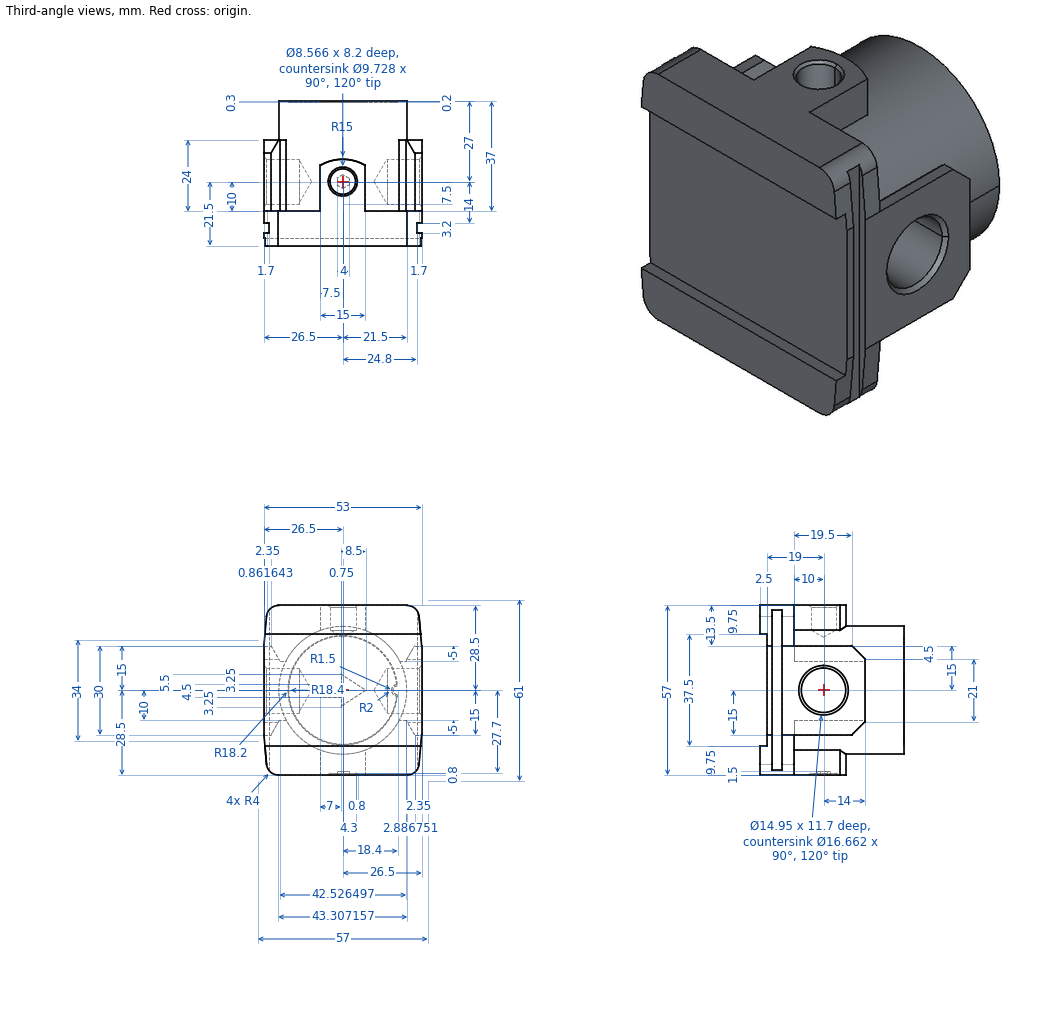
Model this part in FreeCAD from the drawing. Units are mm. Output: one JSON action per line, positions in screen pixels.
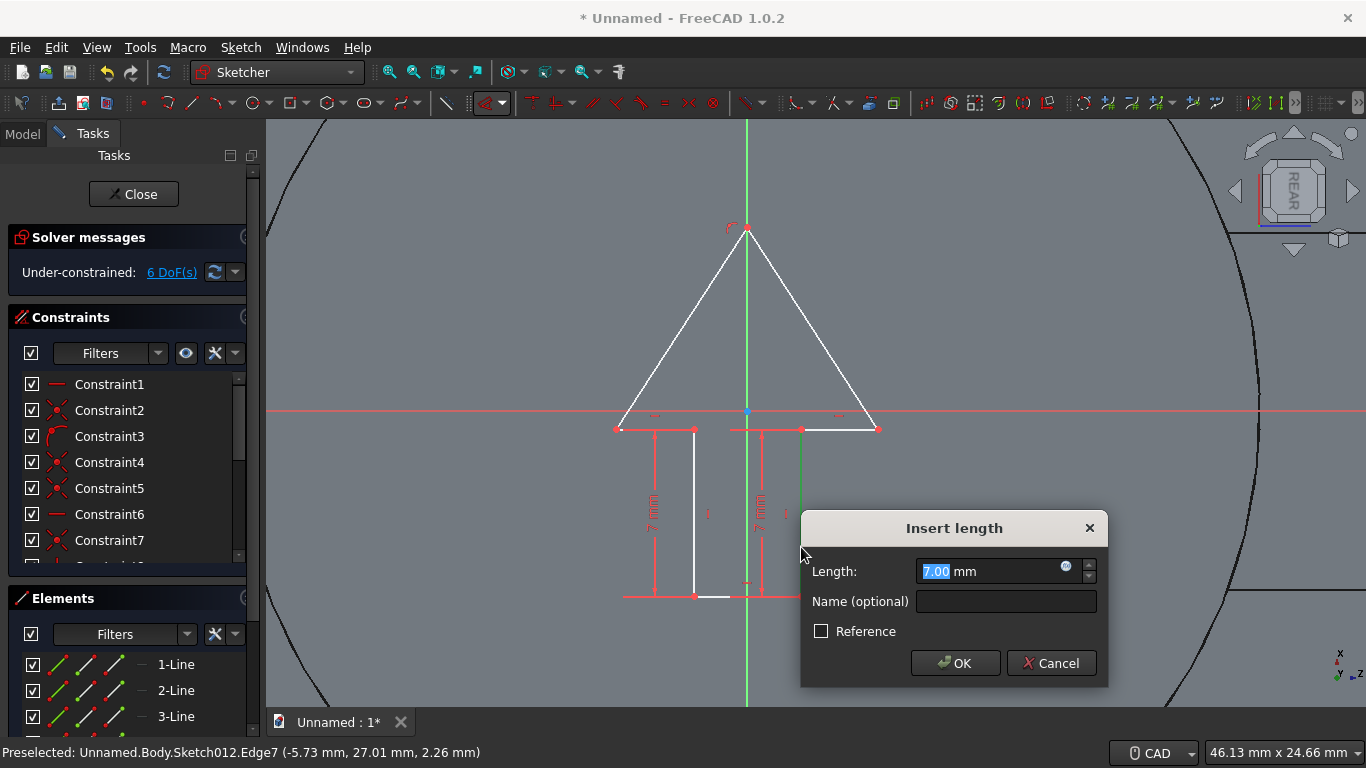
{"action": "type", "text": "7"}
{"action": "key", "text": "Return"}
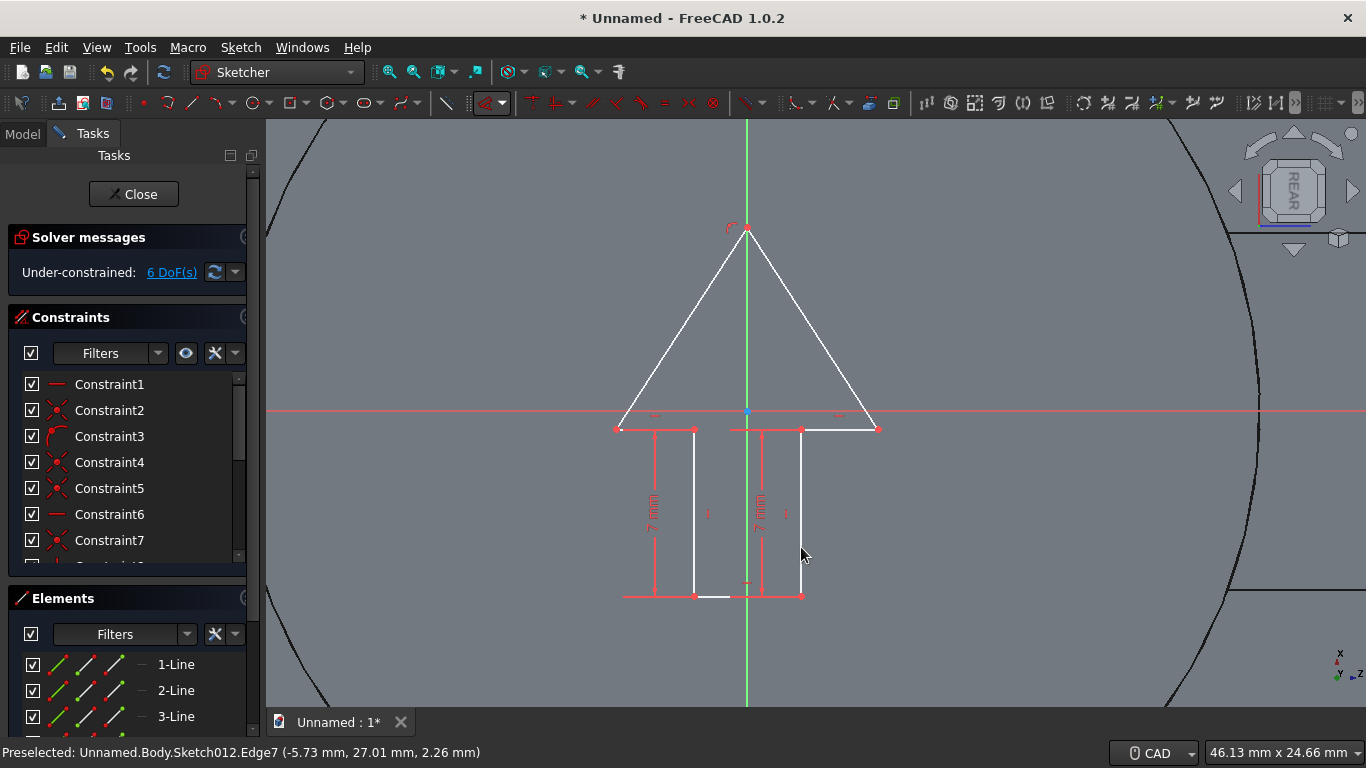
{"action": "left_click", "coordinate": [726, 597]}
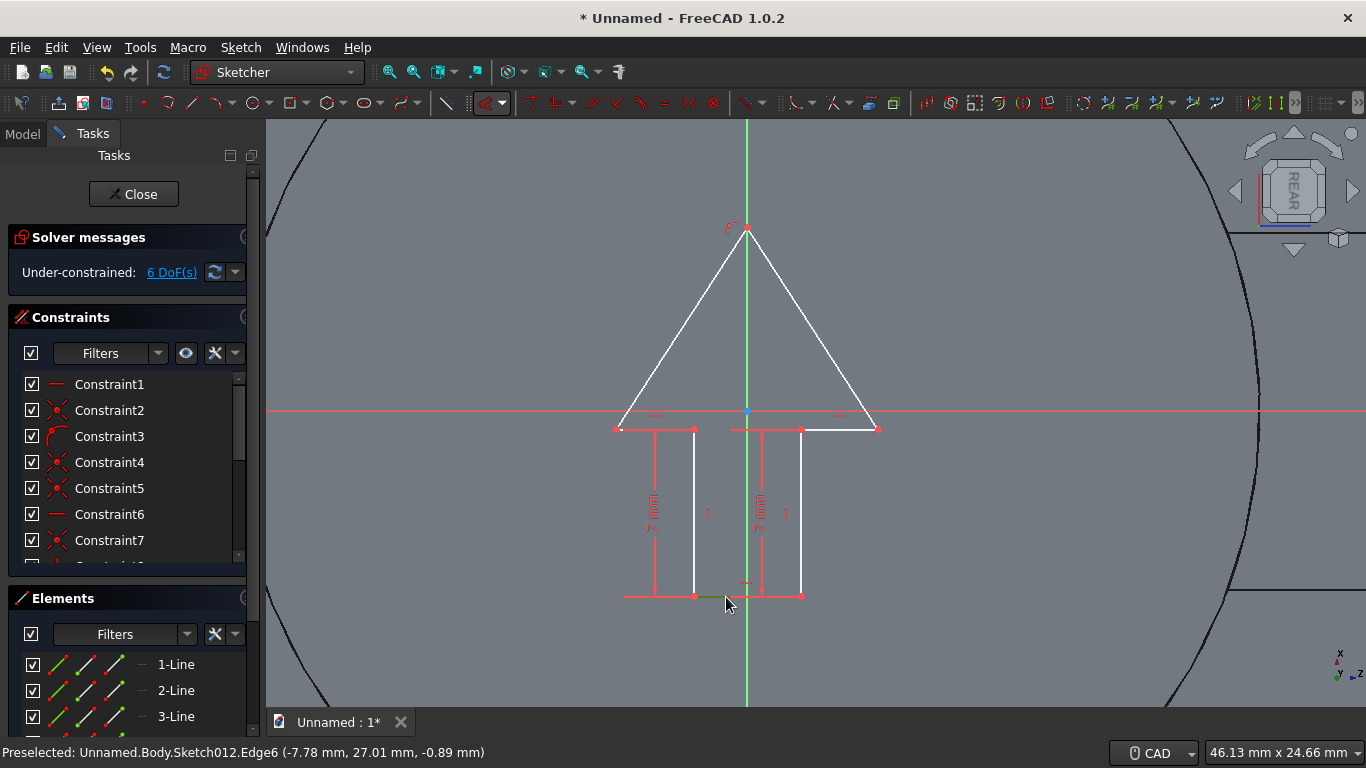
{"action": "key", "text": "l"}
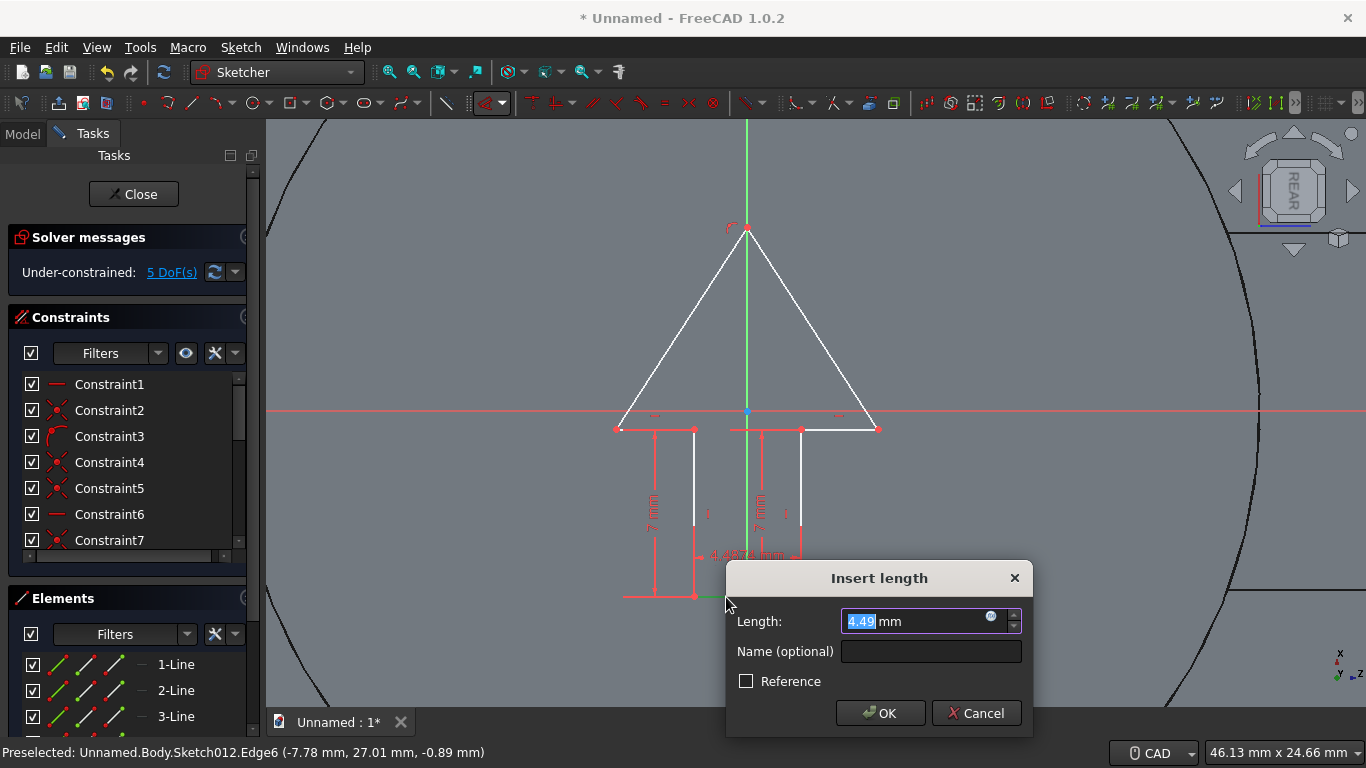
{"action": "type", "text": "4.5"}
{"action": "key", "text": "Return"}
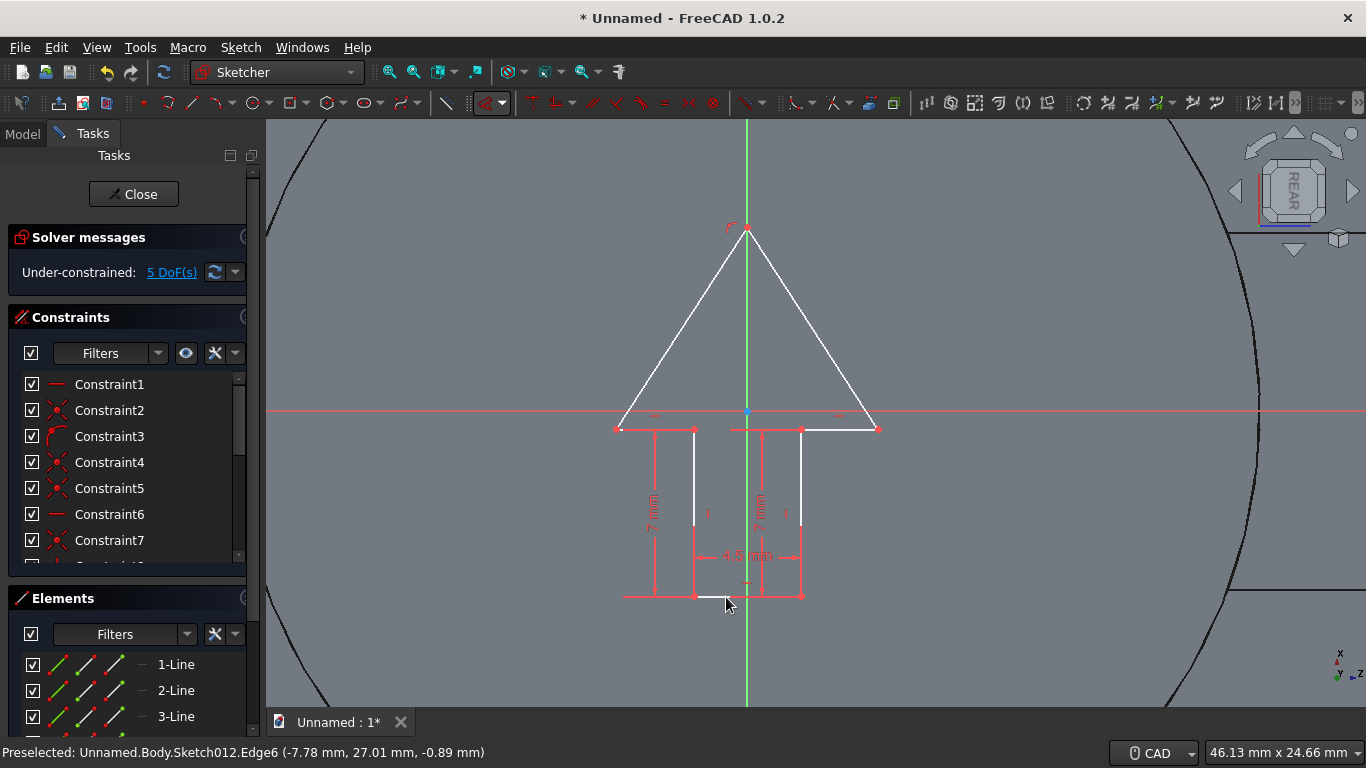
{"action": "left_click", "coordinate": [824, 430]}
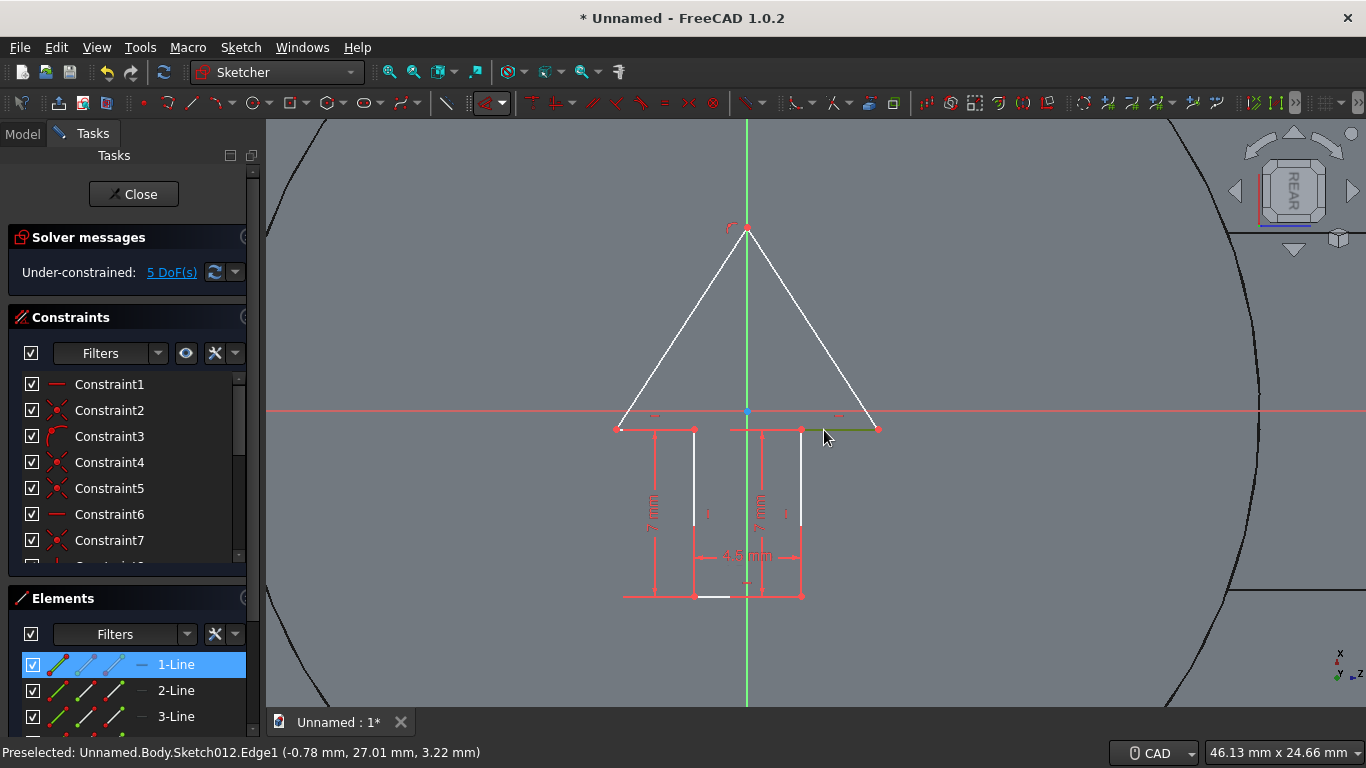
{"action": "key", "text": "l"}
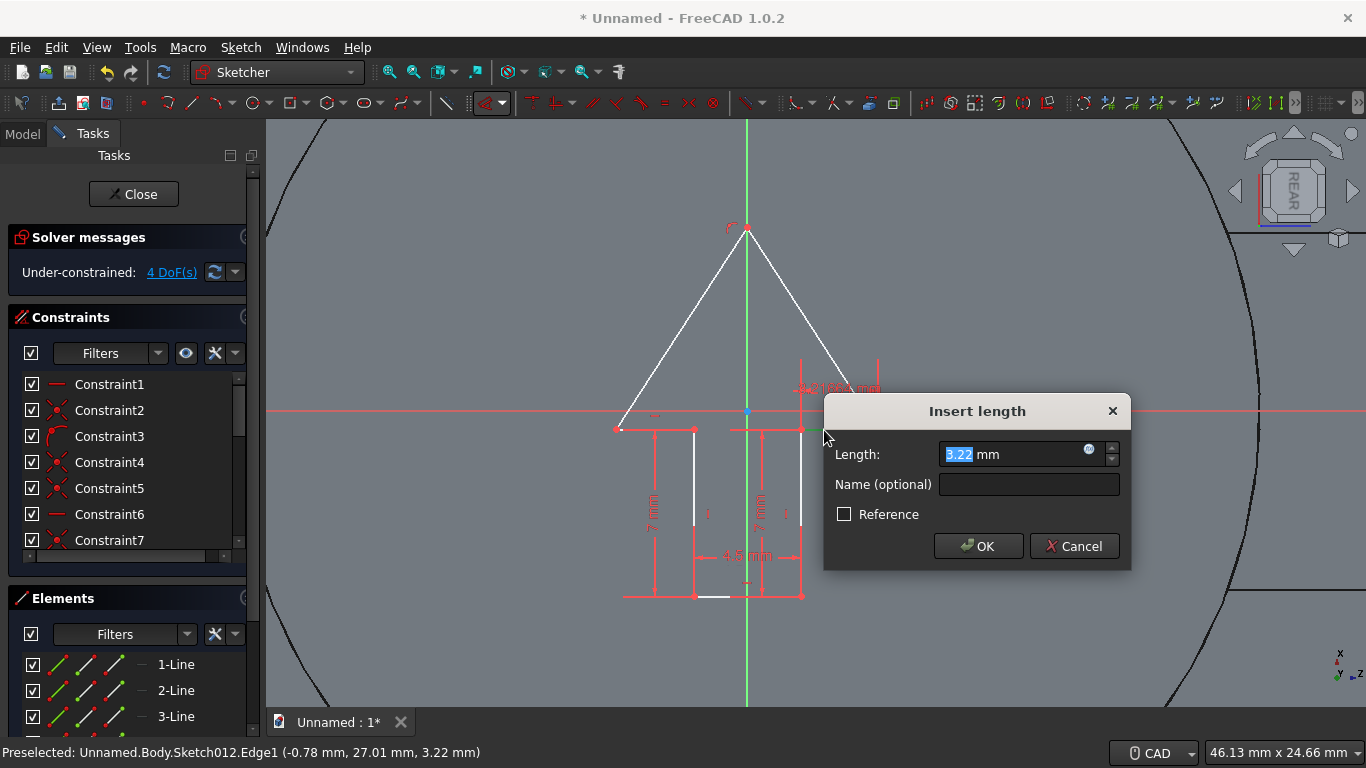
{"action": "type", "text": "3.25"}
{"action": "key", "text": "Return"}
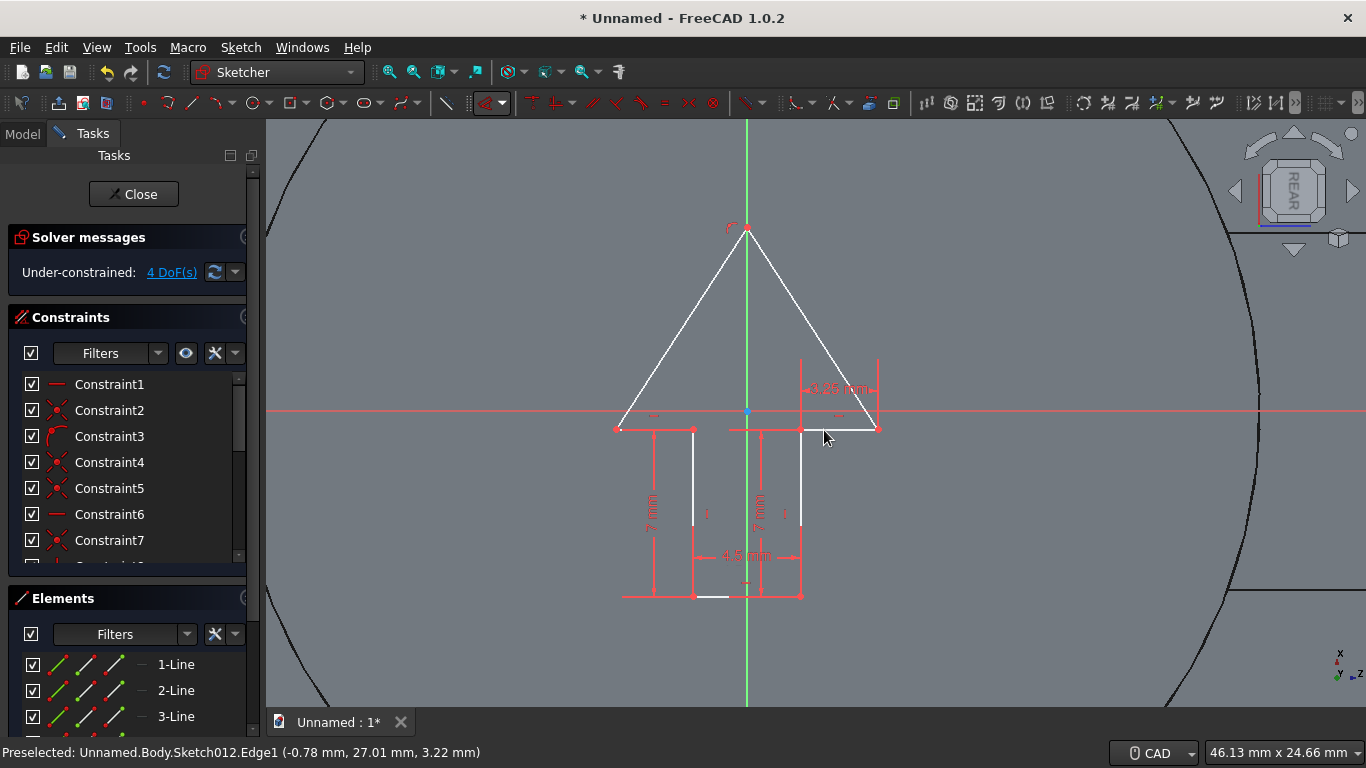
{"action": "left_click", "coordinate": [639, 430]}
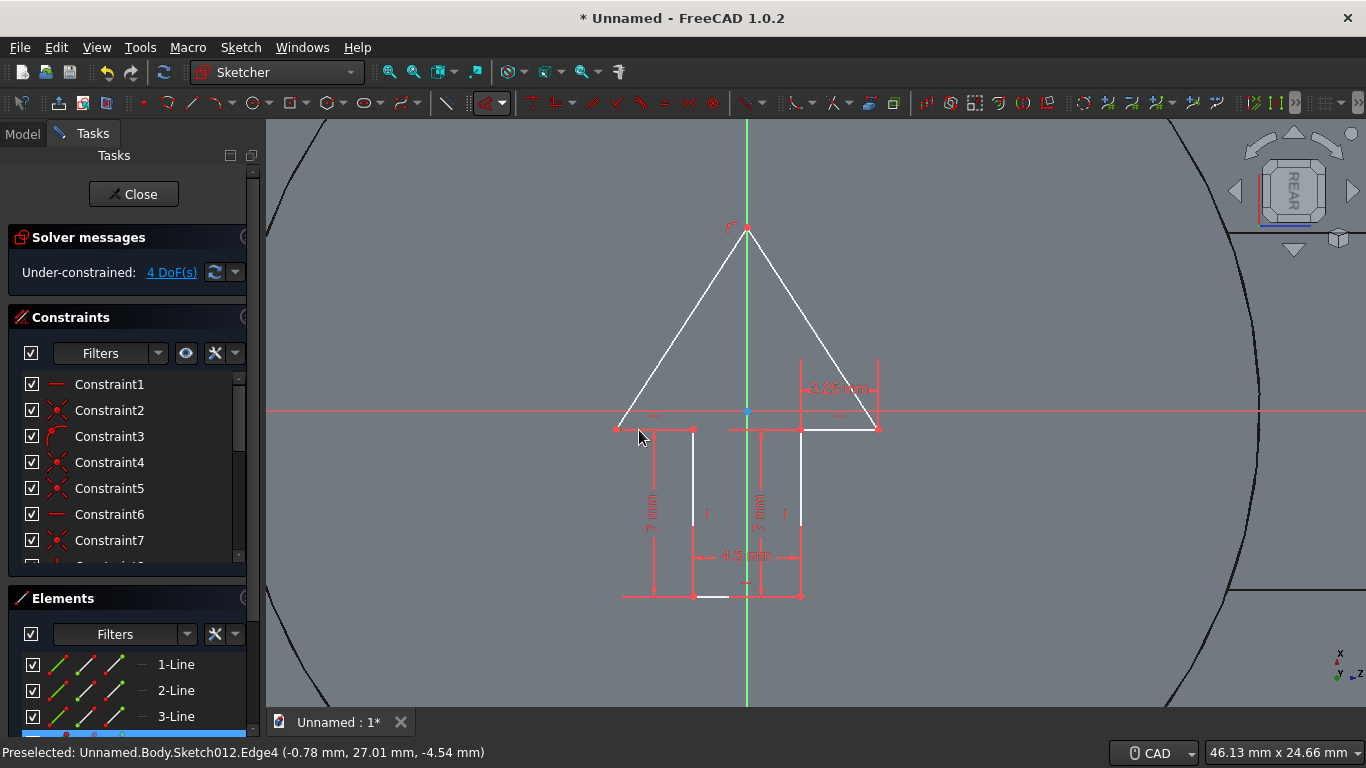
{"action": "left_click", "coordinate": [504, 104]}